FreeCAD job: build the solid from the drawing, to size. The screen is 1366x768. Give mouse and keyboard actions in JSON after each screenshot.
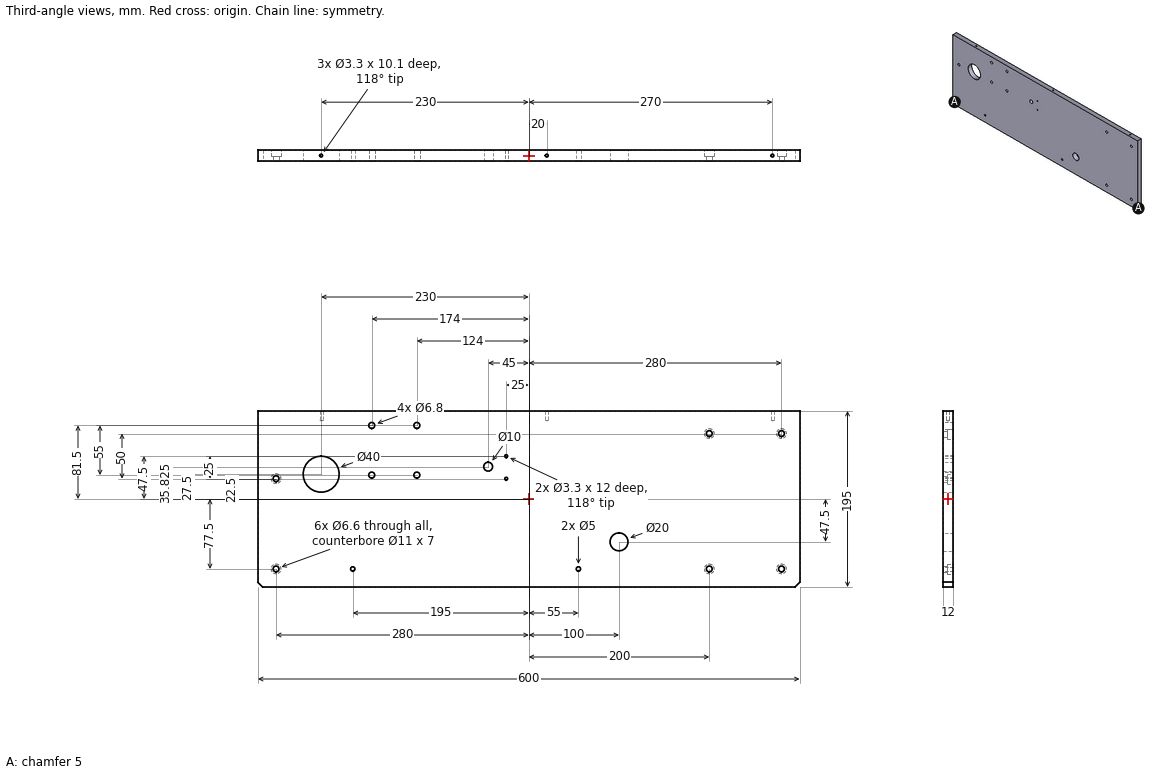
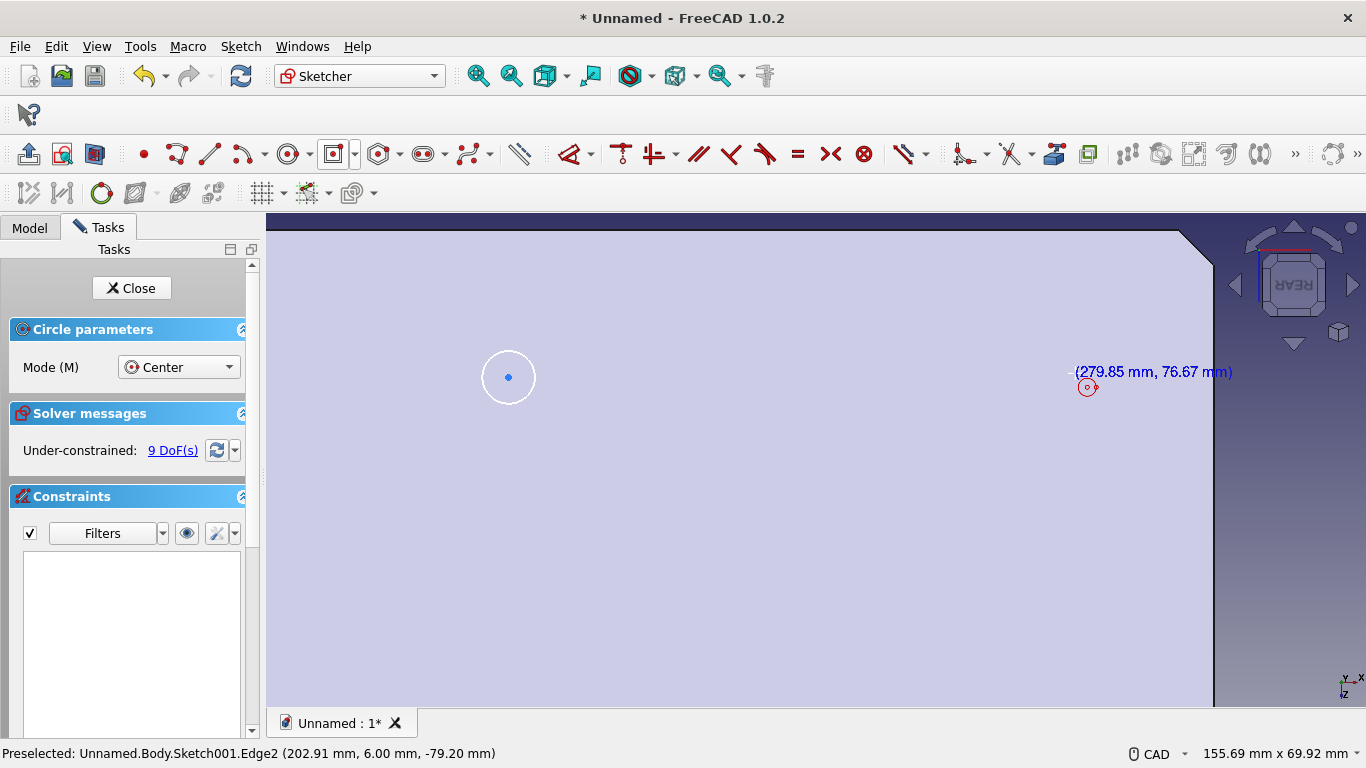
{"action": "scroll", "coordinate": [1075, 373], "scroll_direction": "down", "scroll_amount": 9}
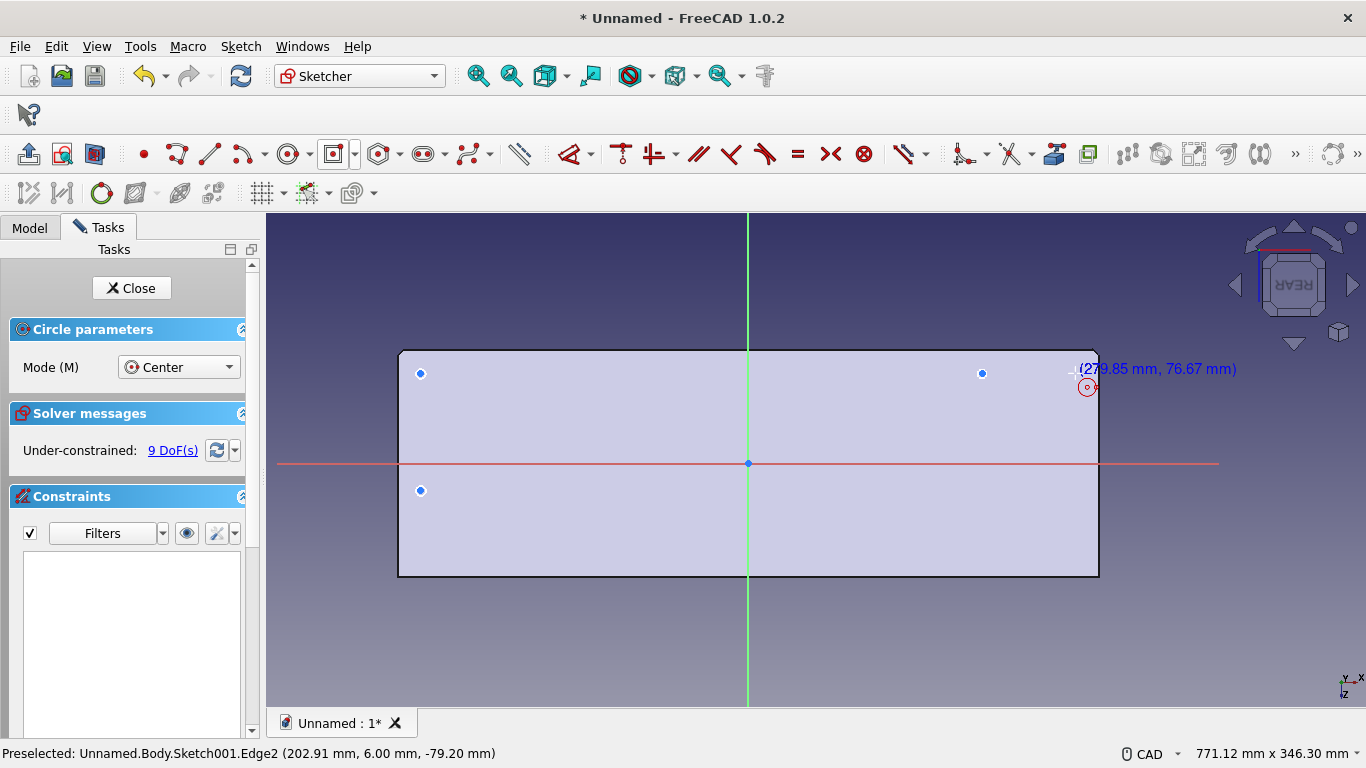
{"action": "left_click", "coordinate": [1075, 373]}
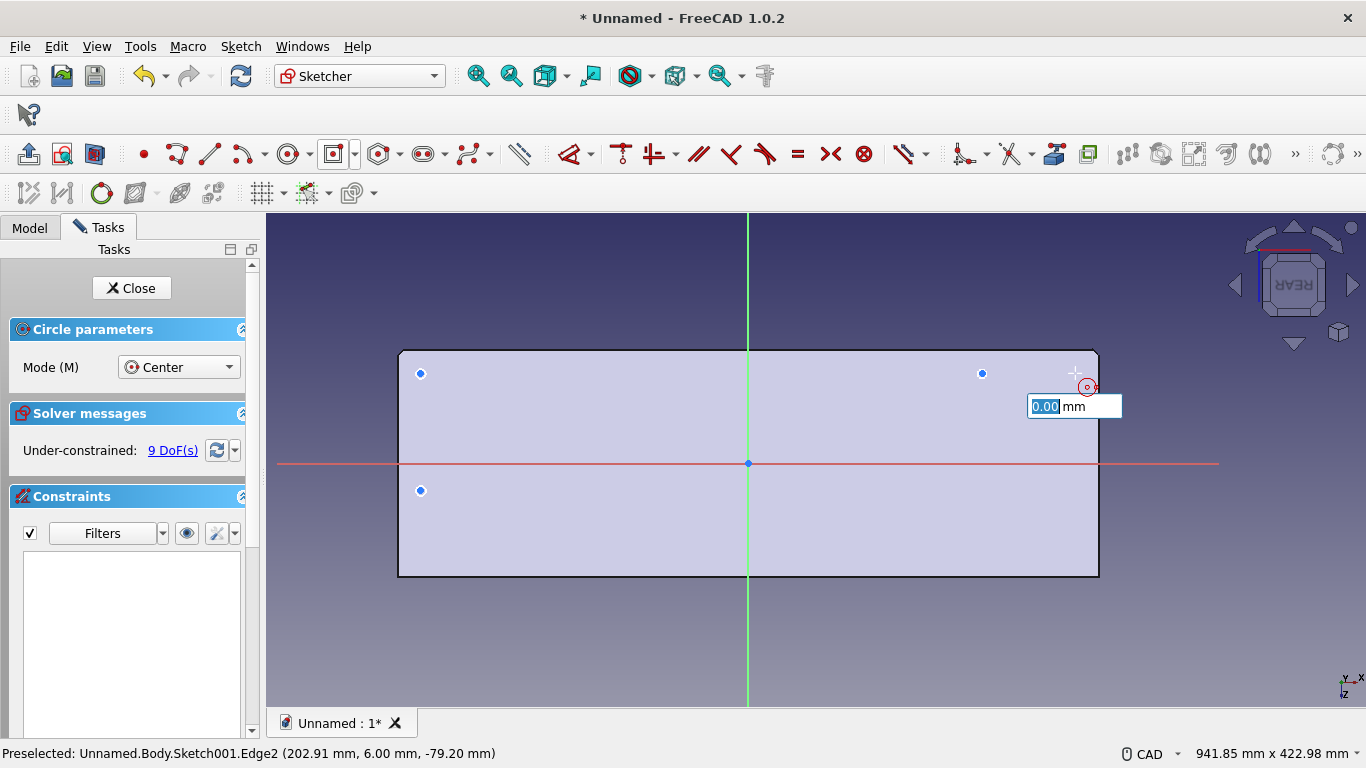
{"action": "scroll", "coordinate": [1078, 370], "scroll_direction": "up", "scroll_amount": 8}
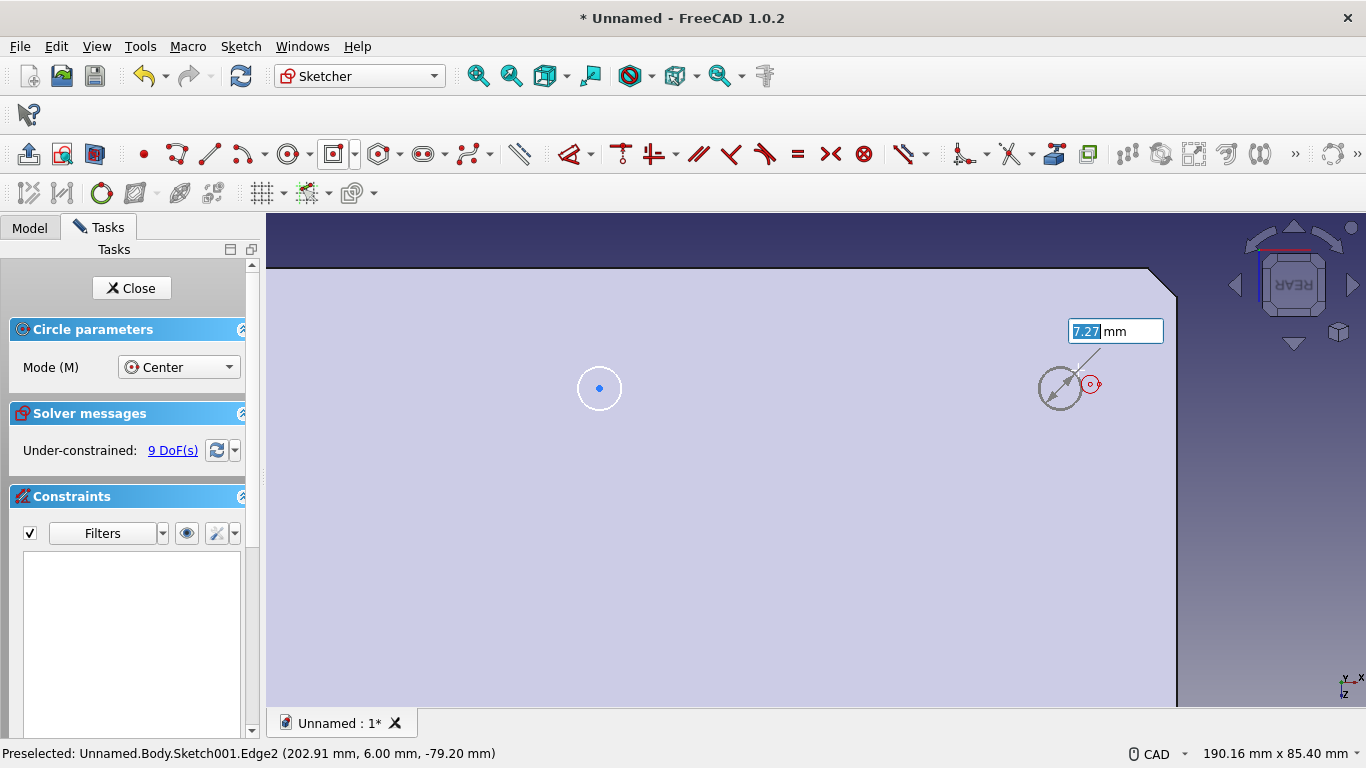
{"action": "left_click", "coordinate": [1075, 370]}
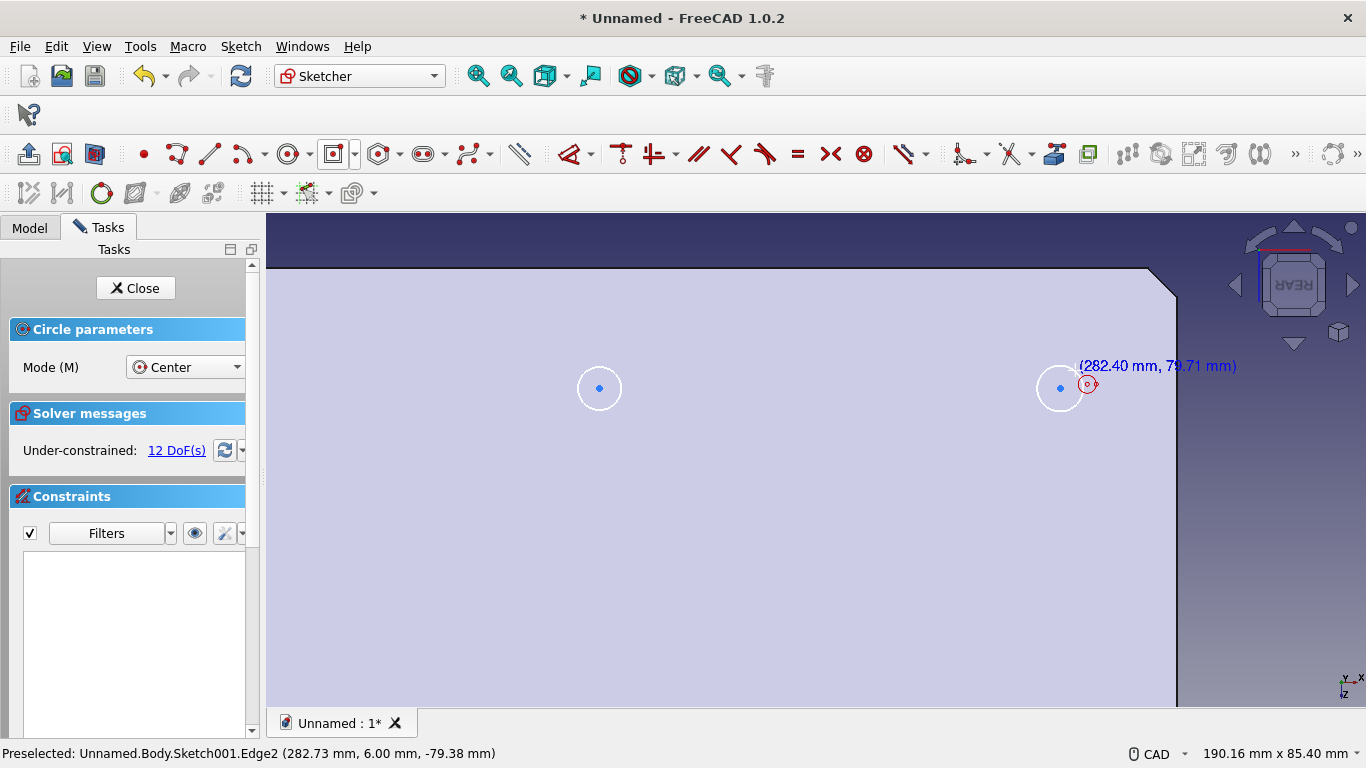
{"action": "scroll", "coordinate": [1078, 370], "scroll_direction": "down", "scroll_amount": 8}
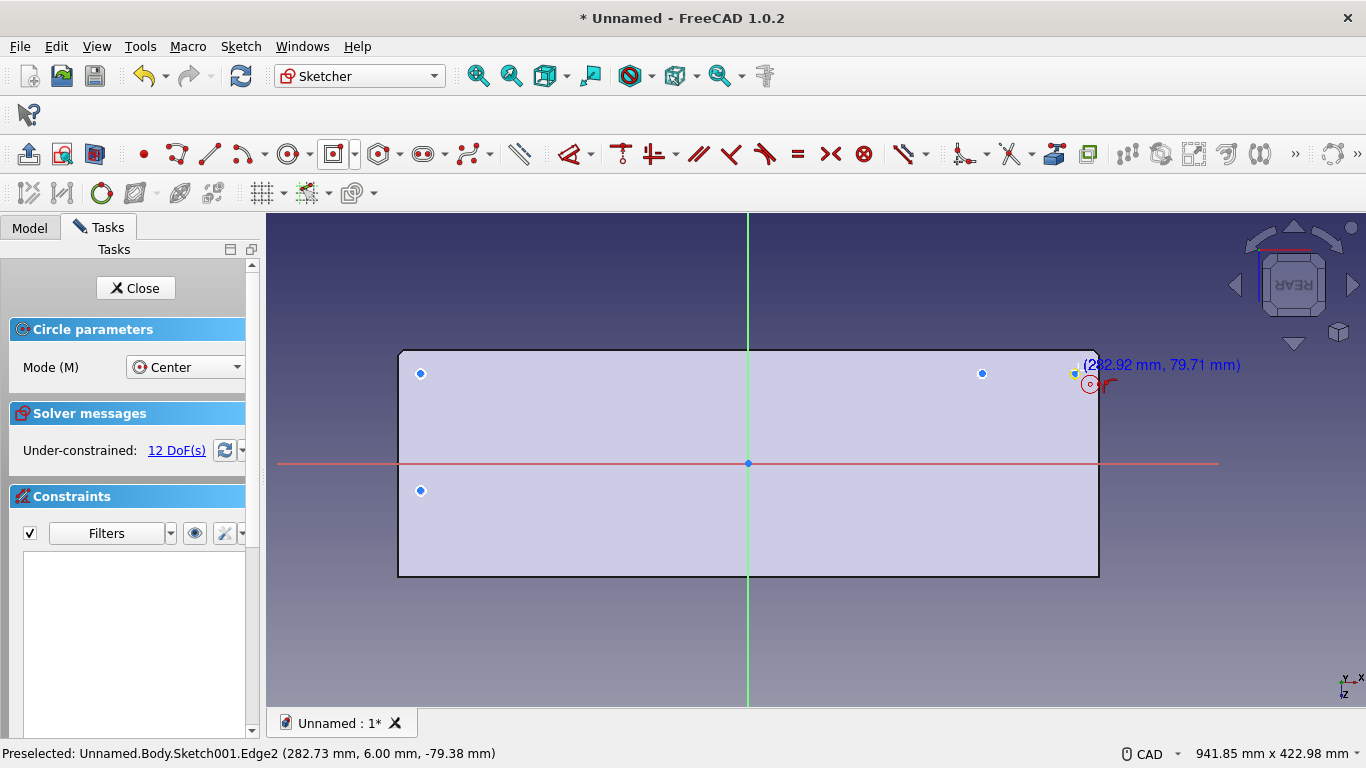
{"action": "scroll", "coordinate": [1075, 548], "scroll_direction": "up", "scroll_amount": 9}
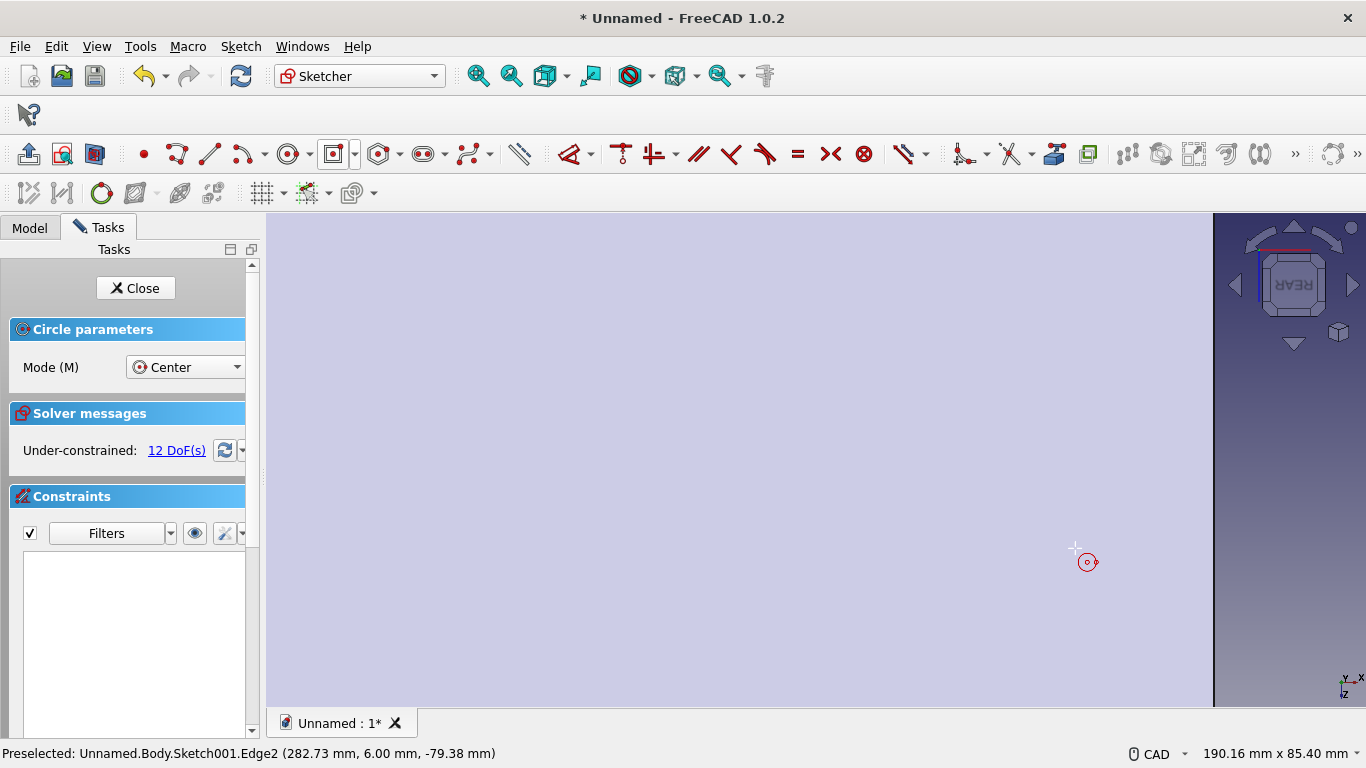
{"action": "scroll", "coordinate": [1075, 548], "scroll_direction": "down", "scroll_amount": 9}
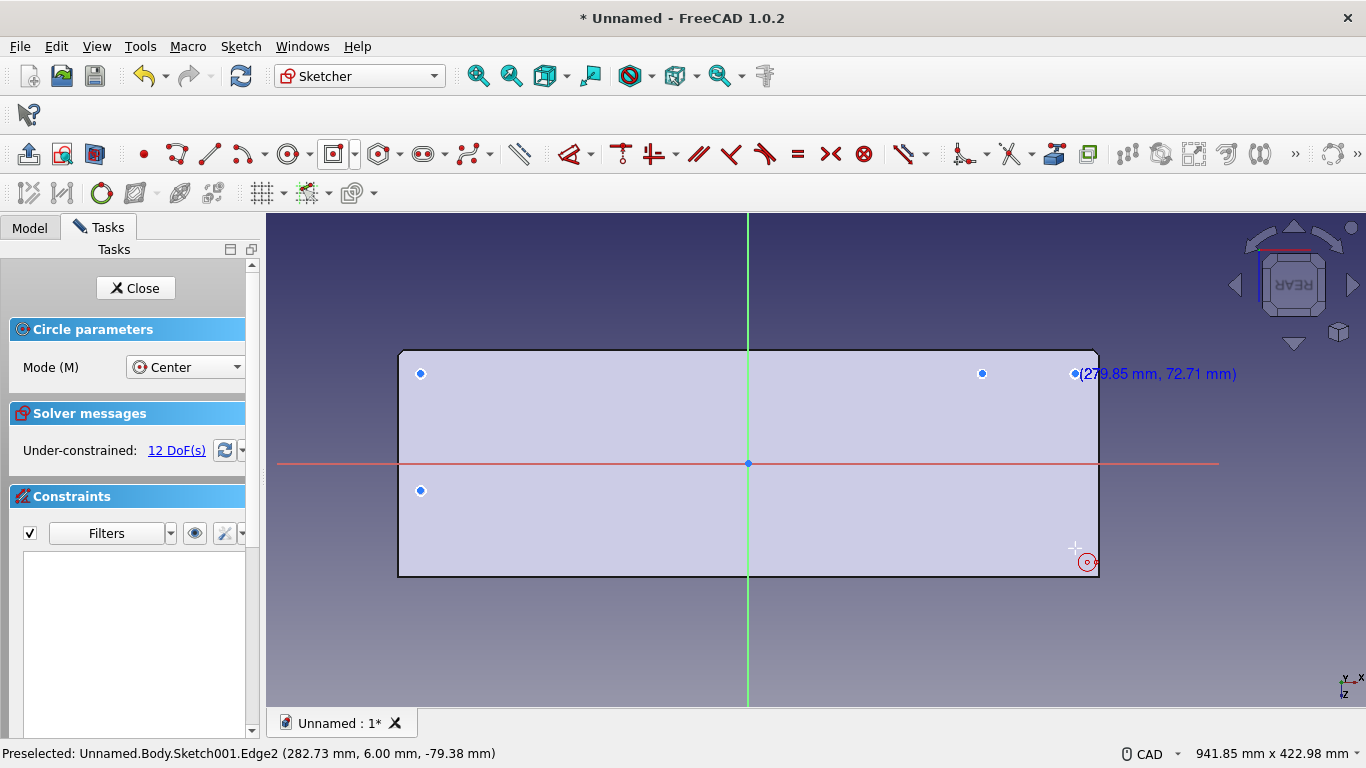
{"action": "left_click", "coordinate": [1075, 548]}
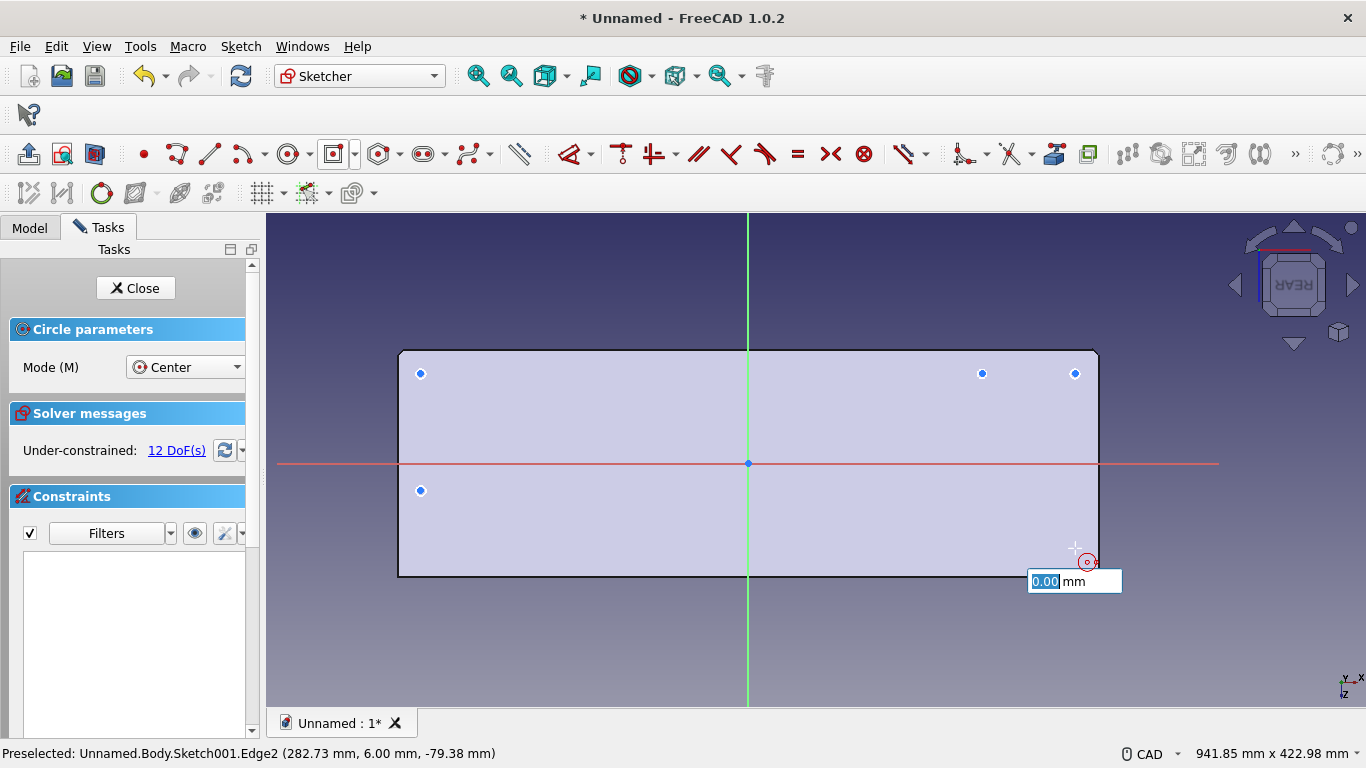
{"action": "scroll", "coordinate": [1078, 545], "scroll_direction": "up", "scroll_amount": 8}